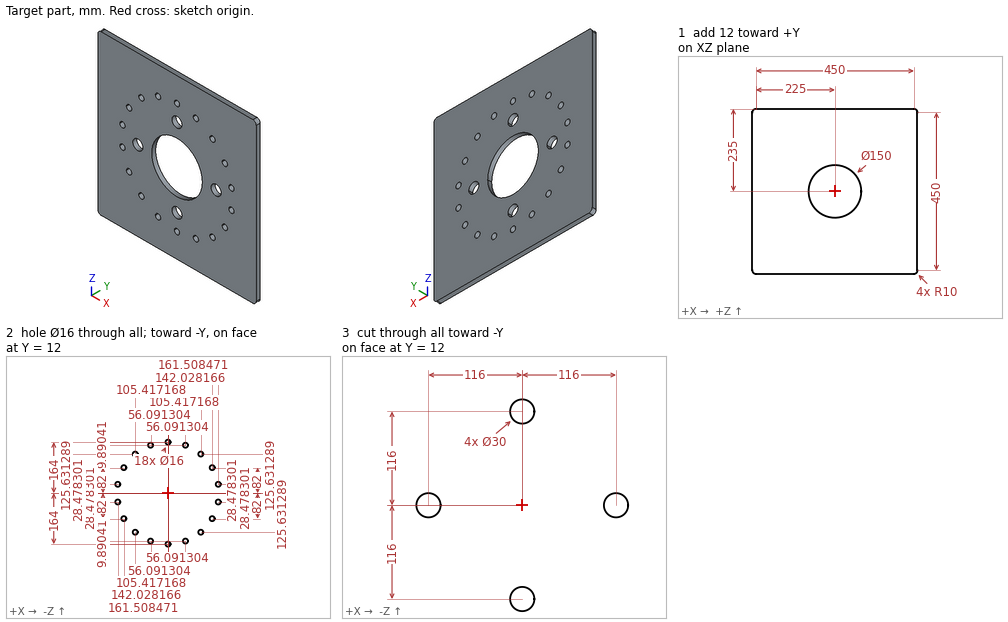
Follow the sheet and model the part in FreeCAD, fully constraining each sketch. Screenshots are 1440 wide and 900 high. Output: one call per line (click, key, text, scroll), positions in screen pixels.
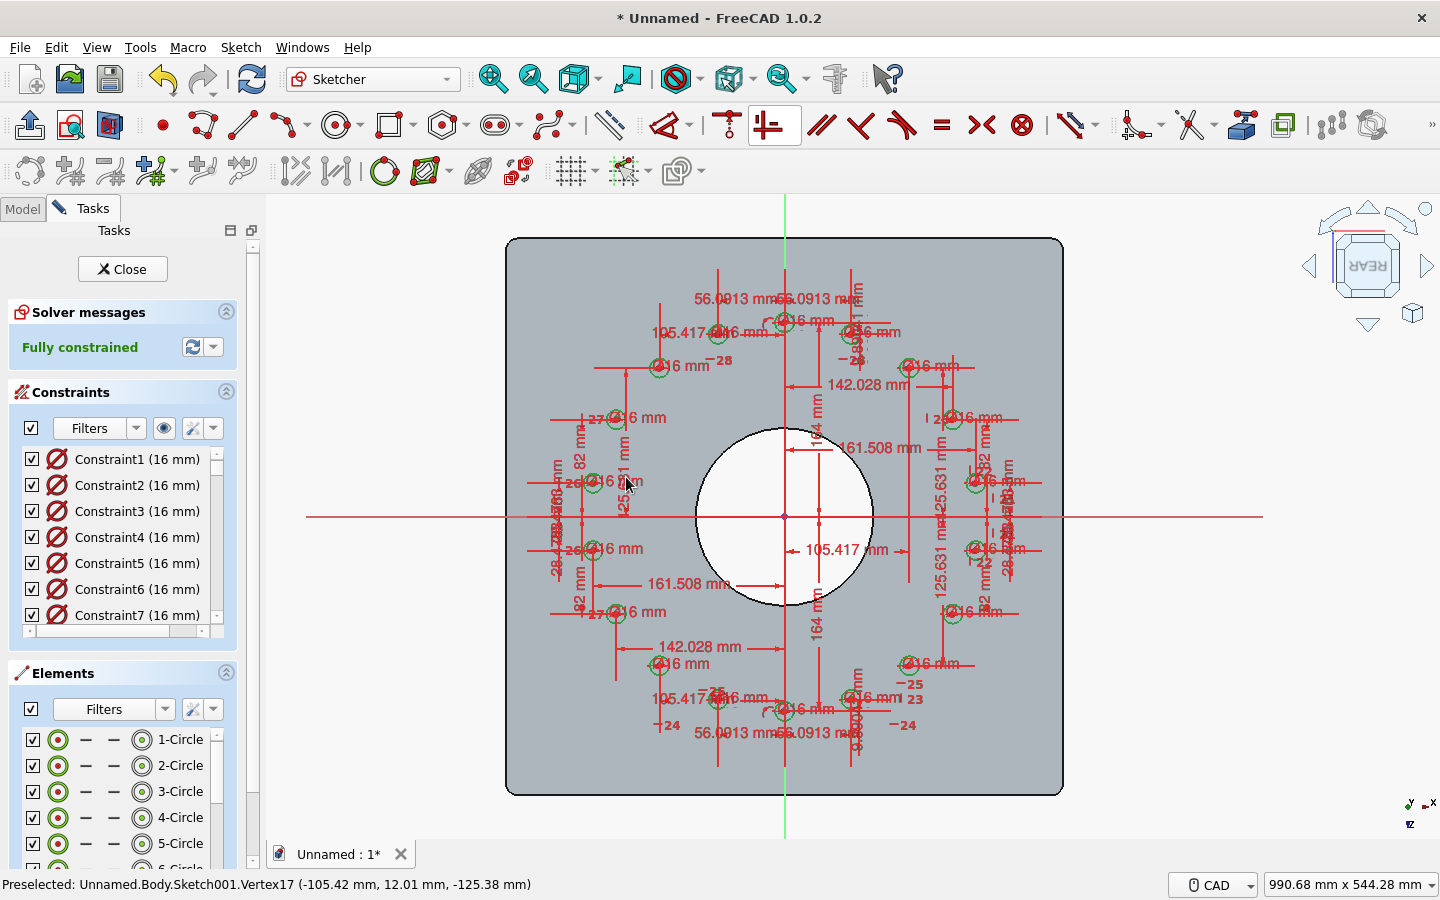
click(123, 269)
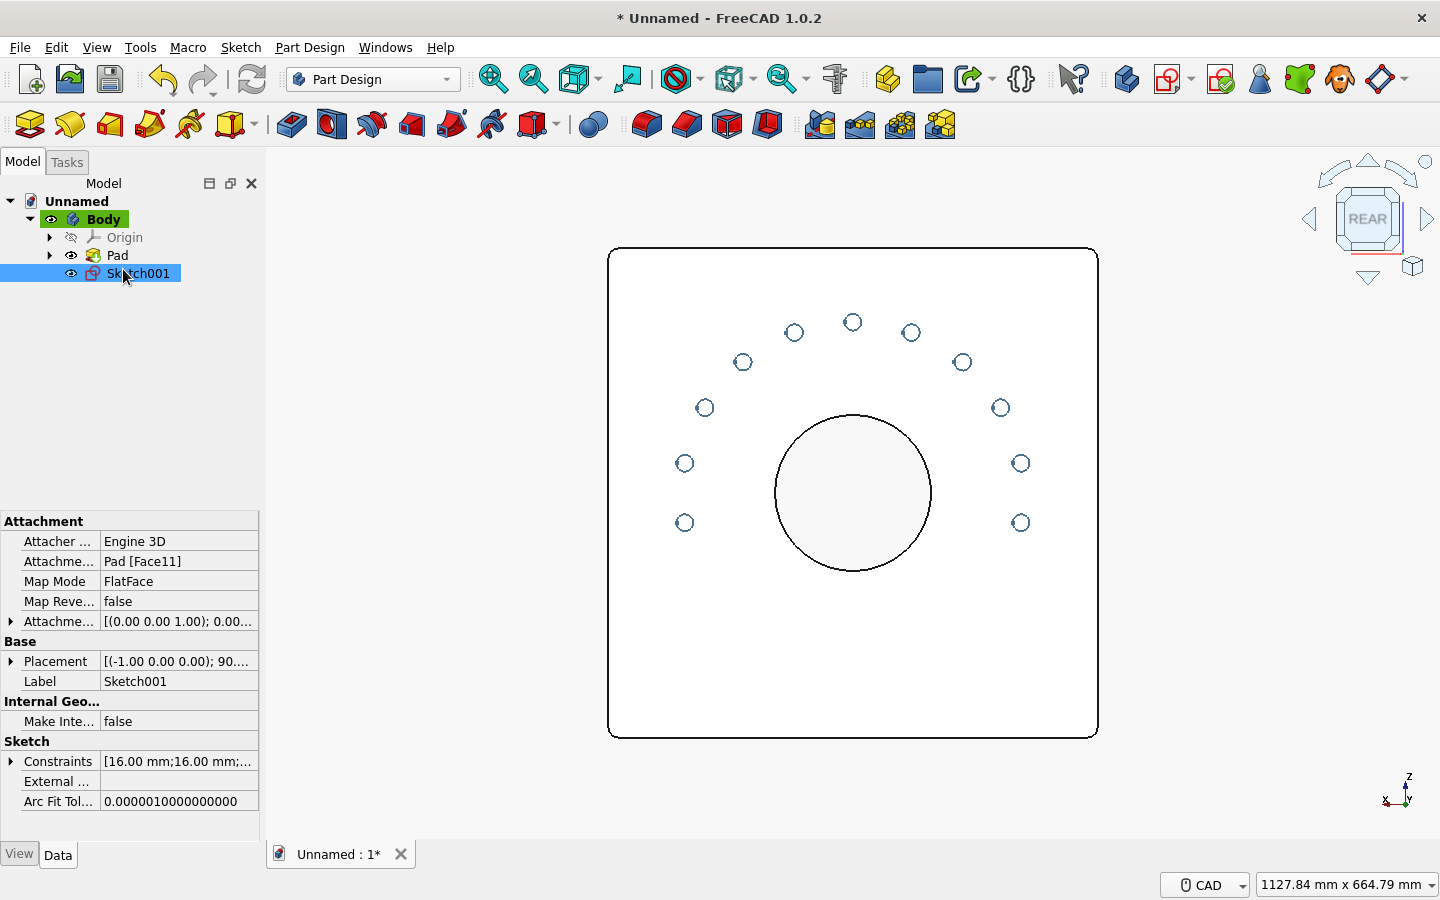
click(332, 124)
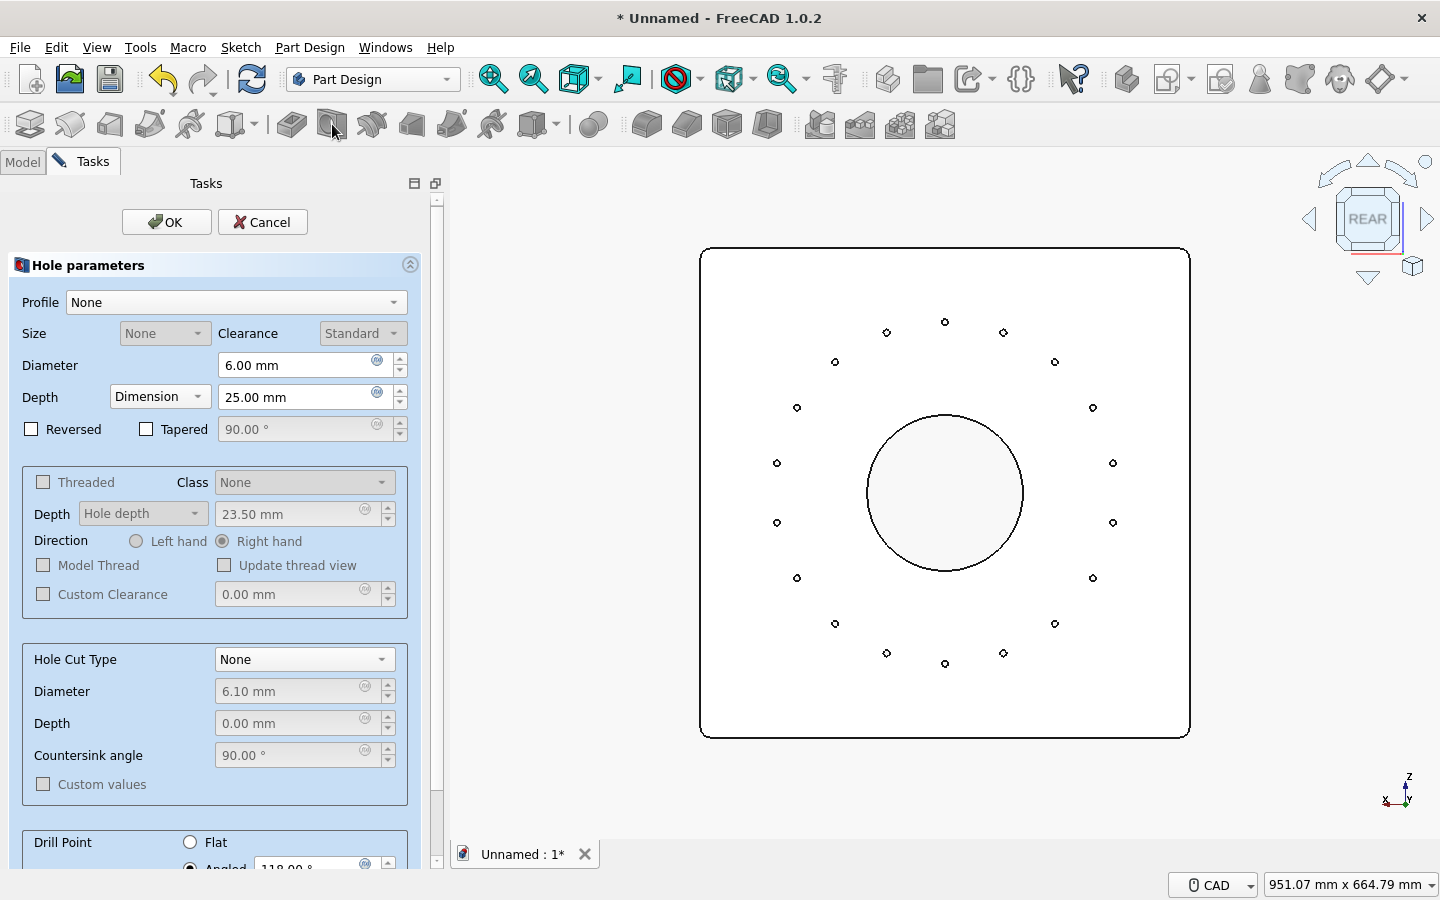
triple_click(305, 365)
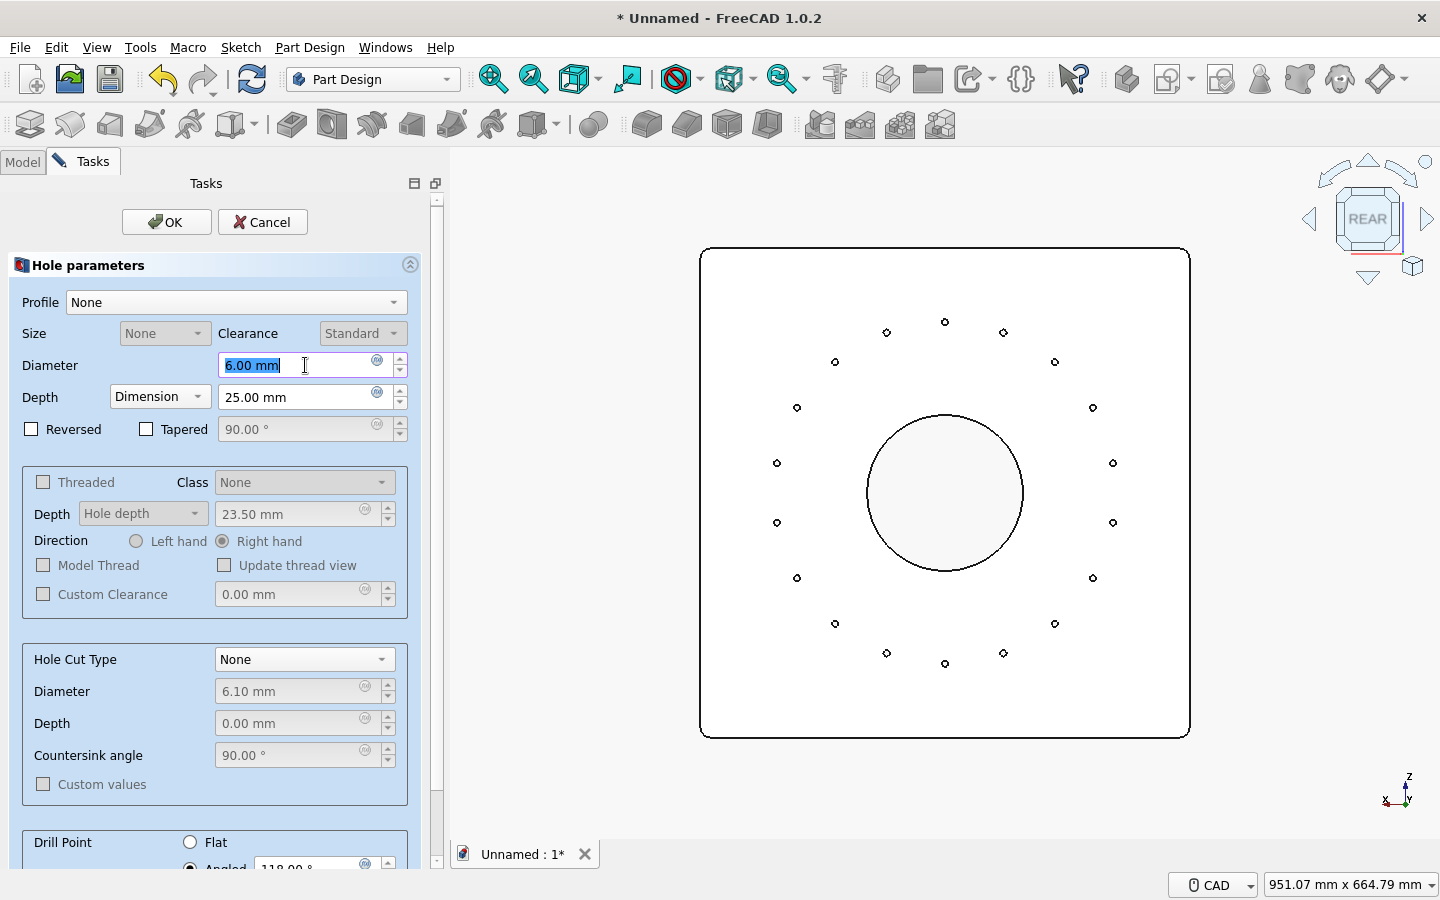
text(16)
key(Tab)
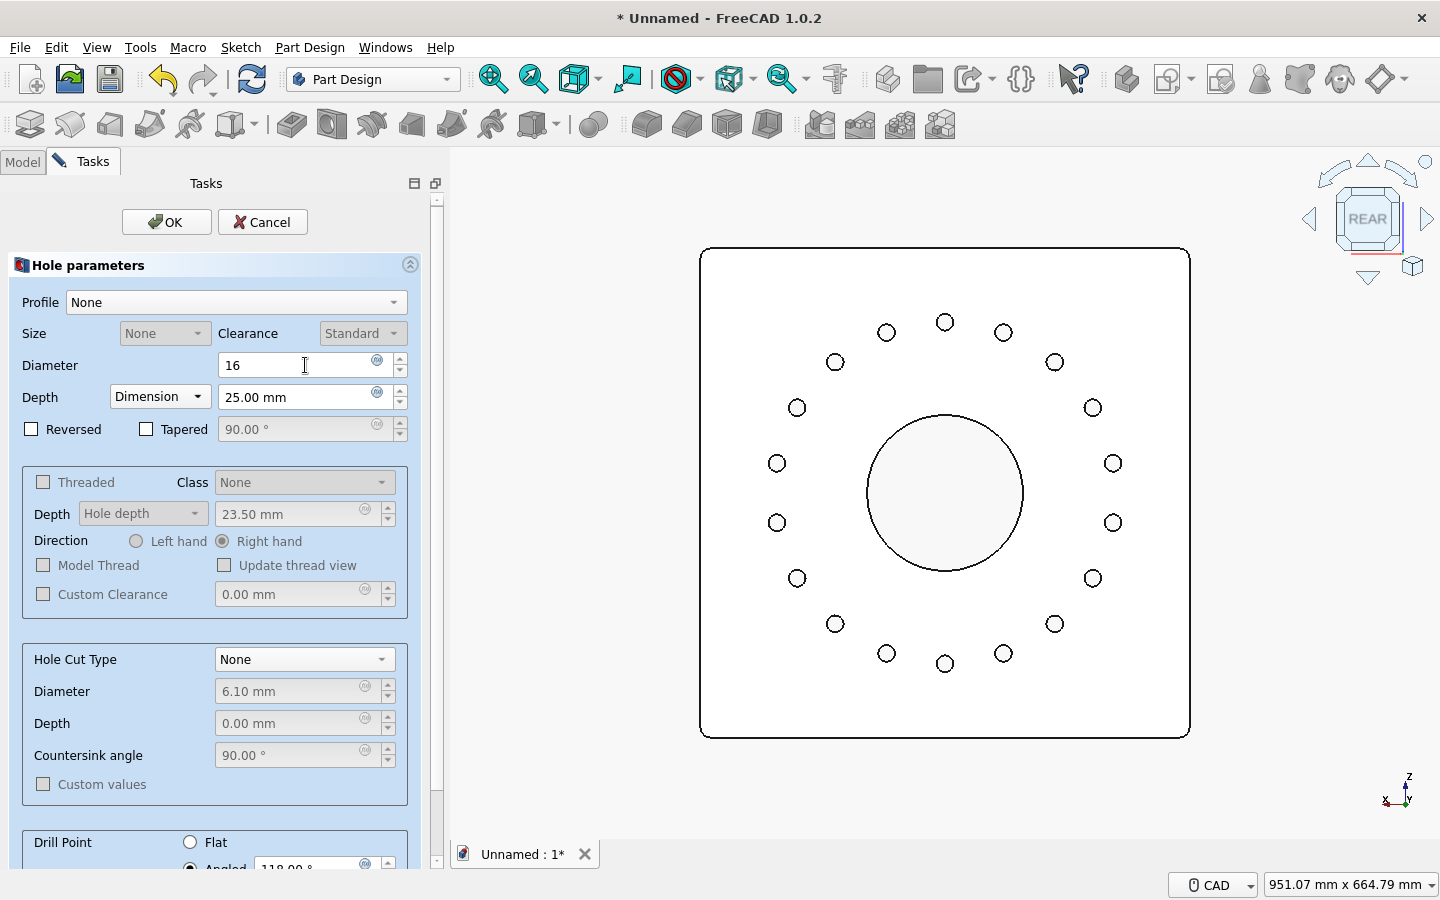
click(161, 396)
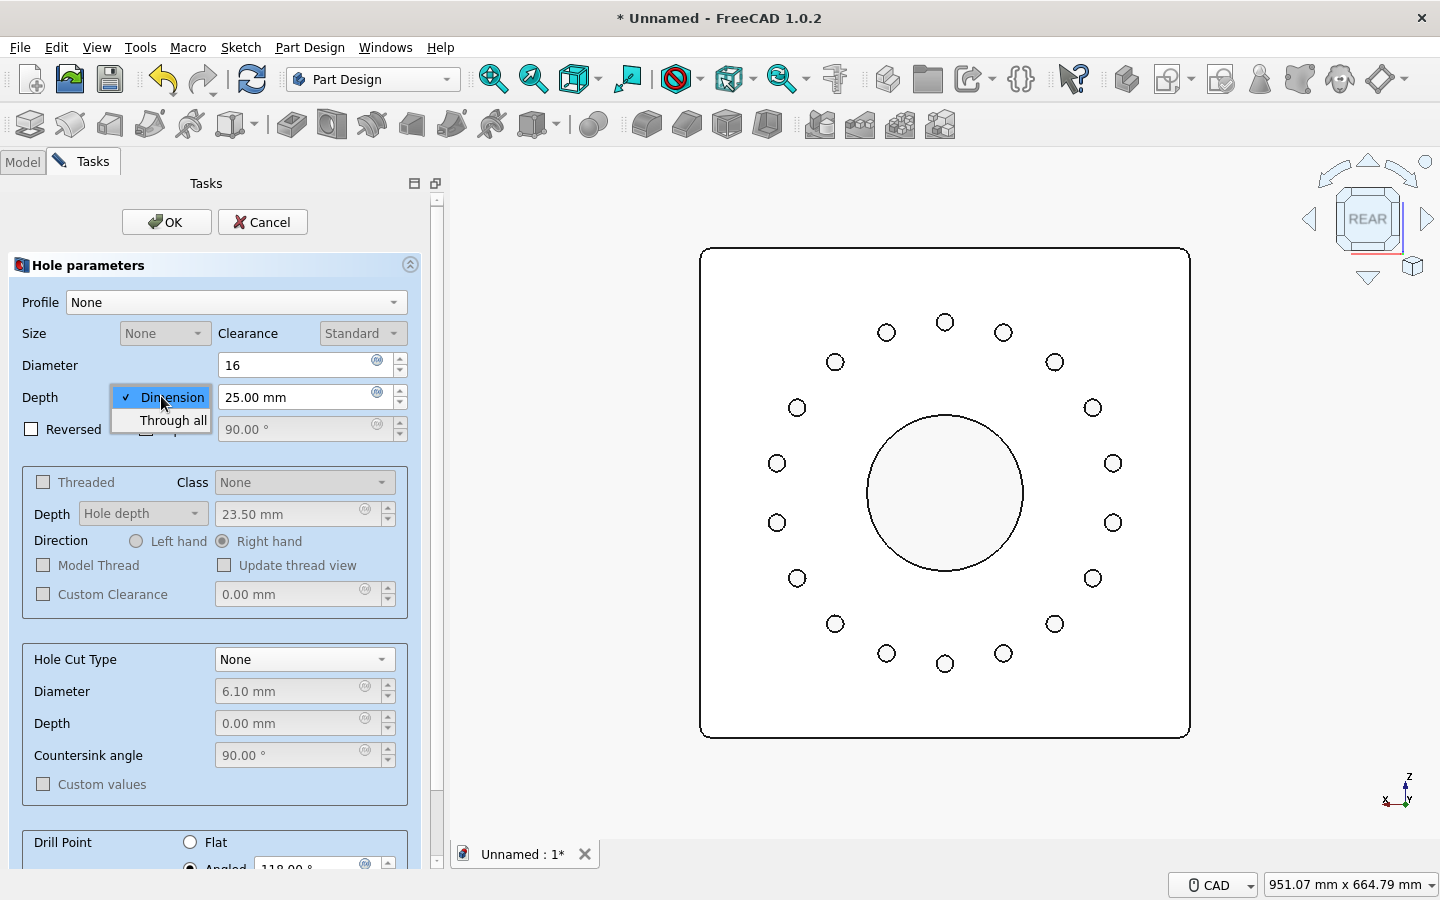
click(160, 420)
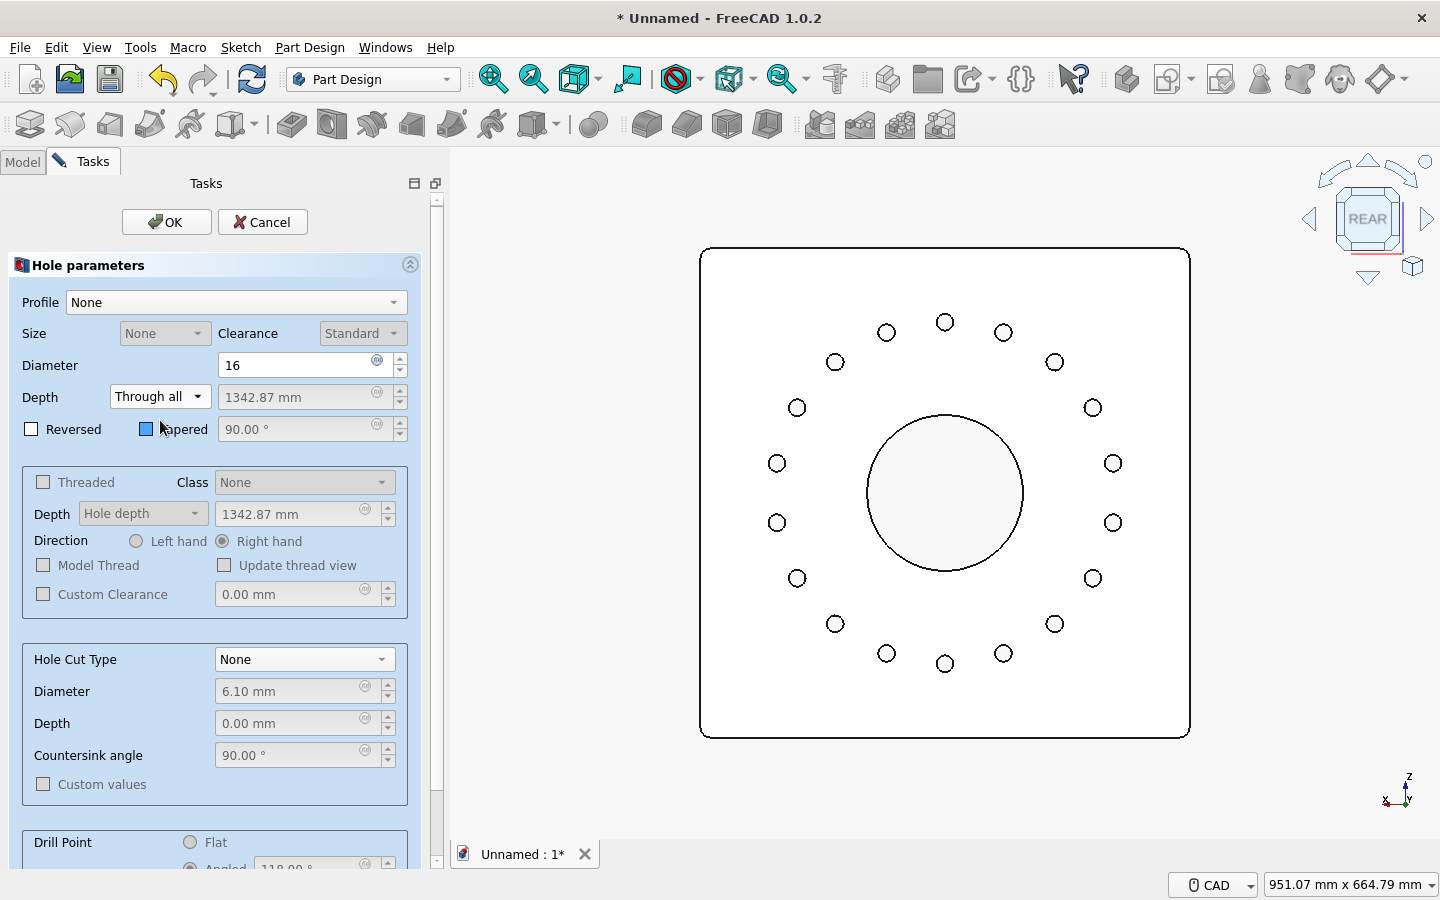
click(167, 222)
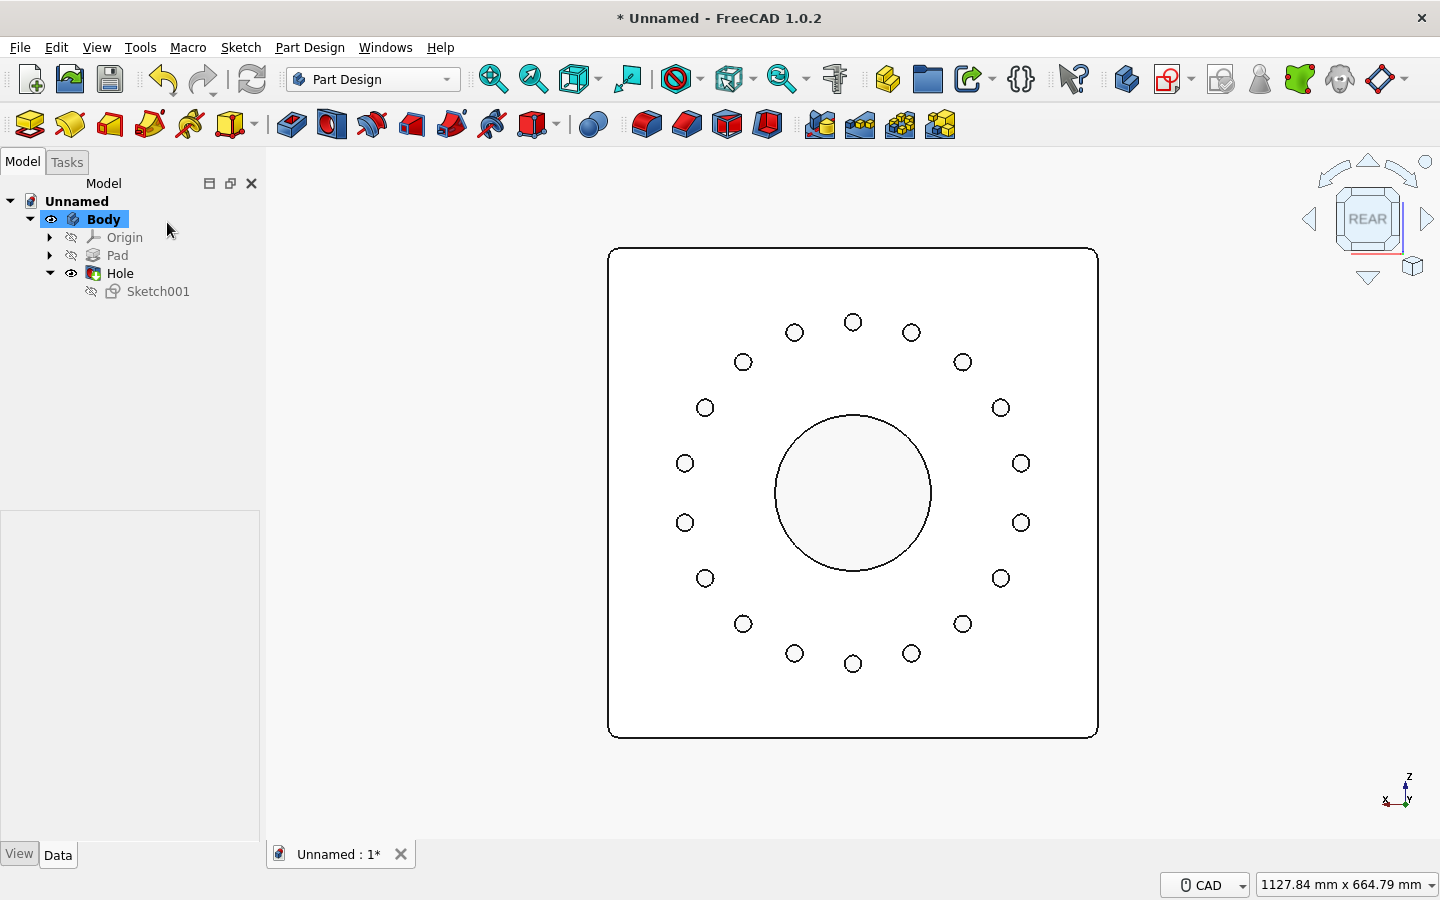
click(643, 352)